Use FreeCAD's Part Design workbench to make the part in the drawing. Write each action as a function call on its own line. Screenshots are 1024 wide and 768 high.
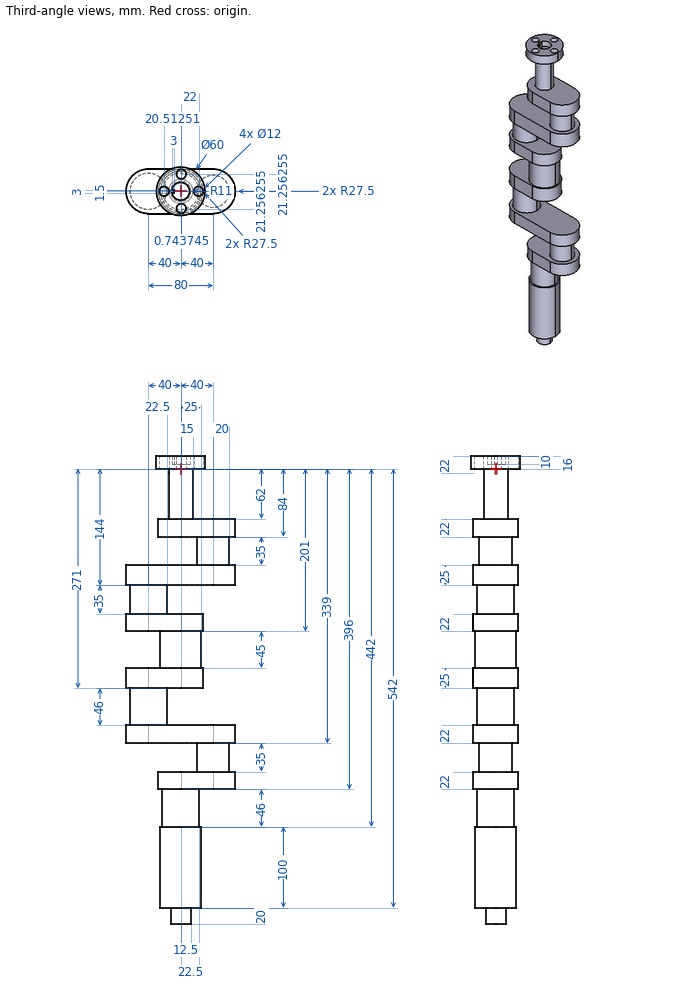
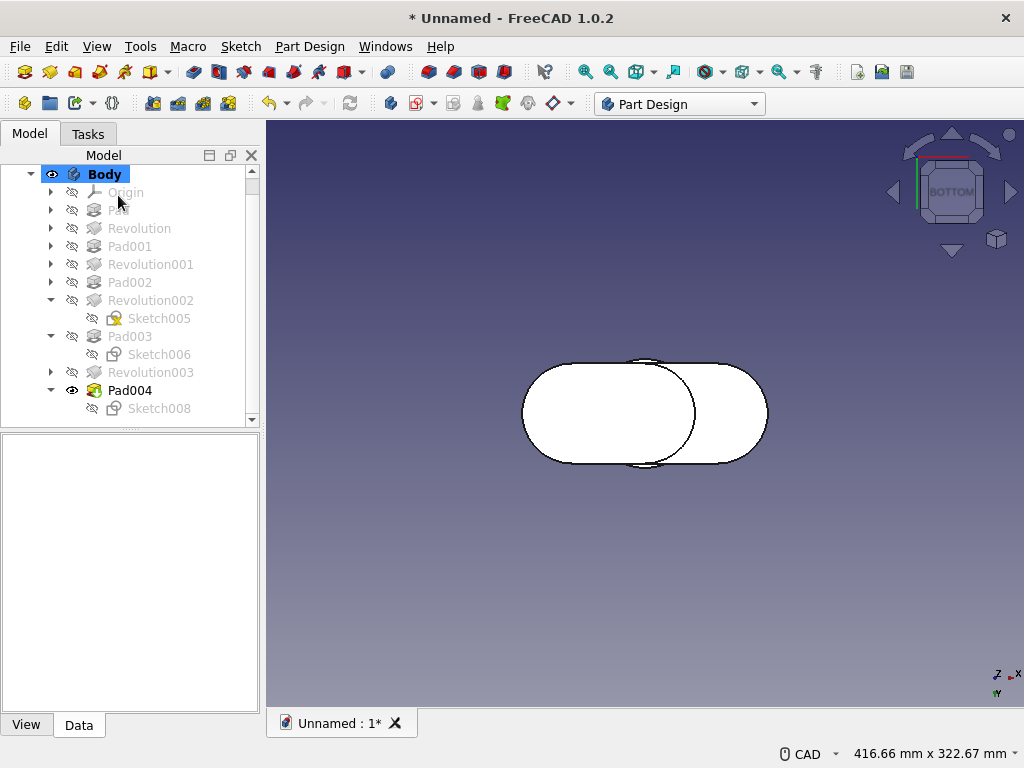
click(416, 104)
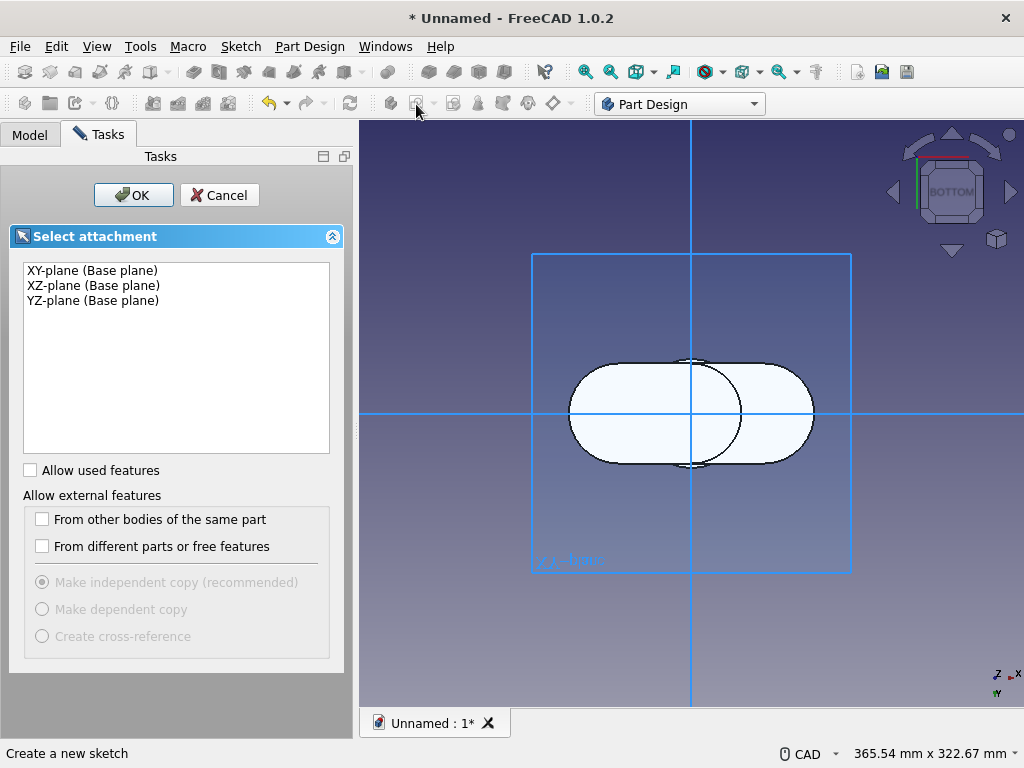
click(84, 286)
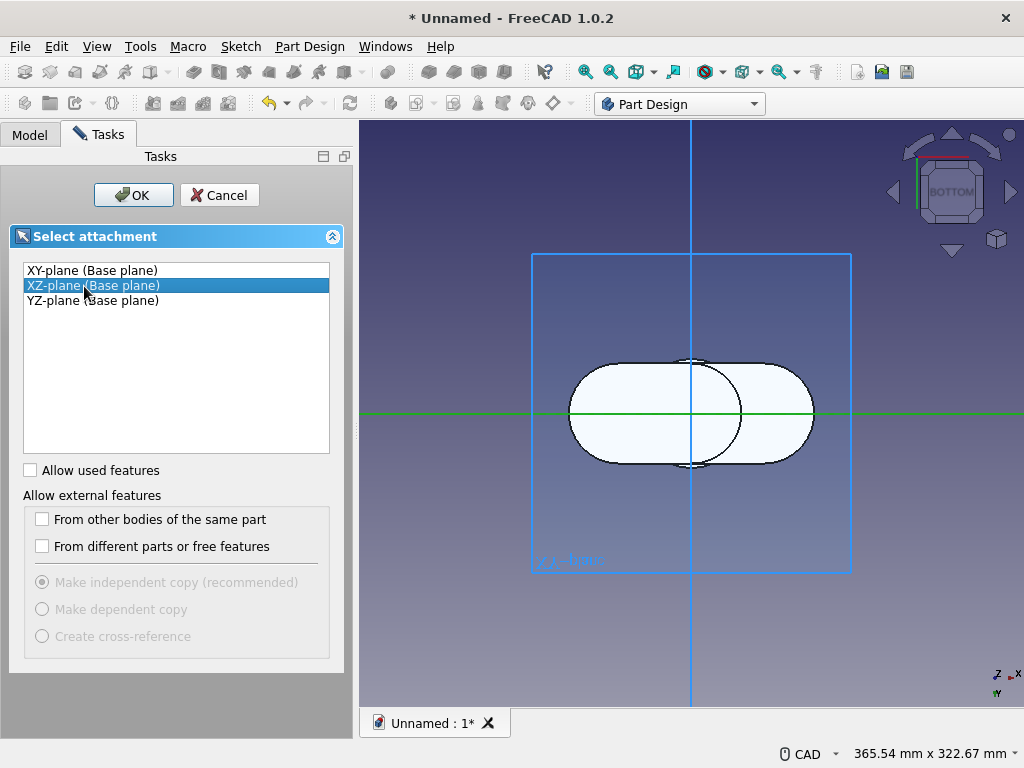
click(134, 195)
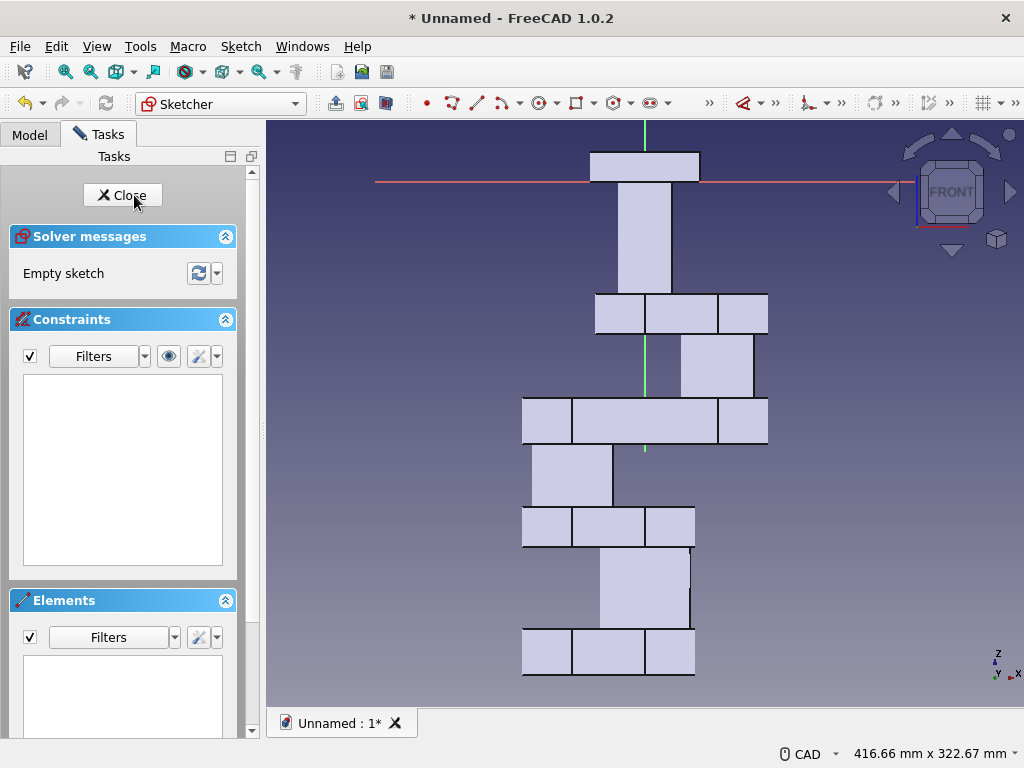
click(386, 104)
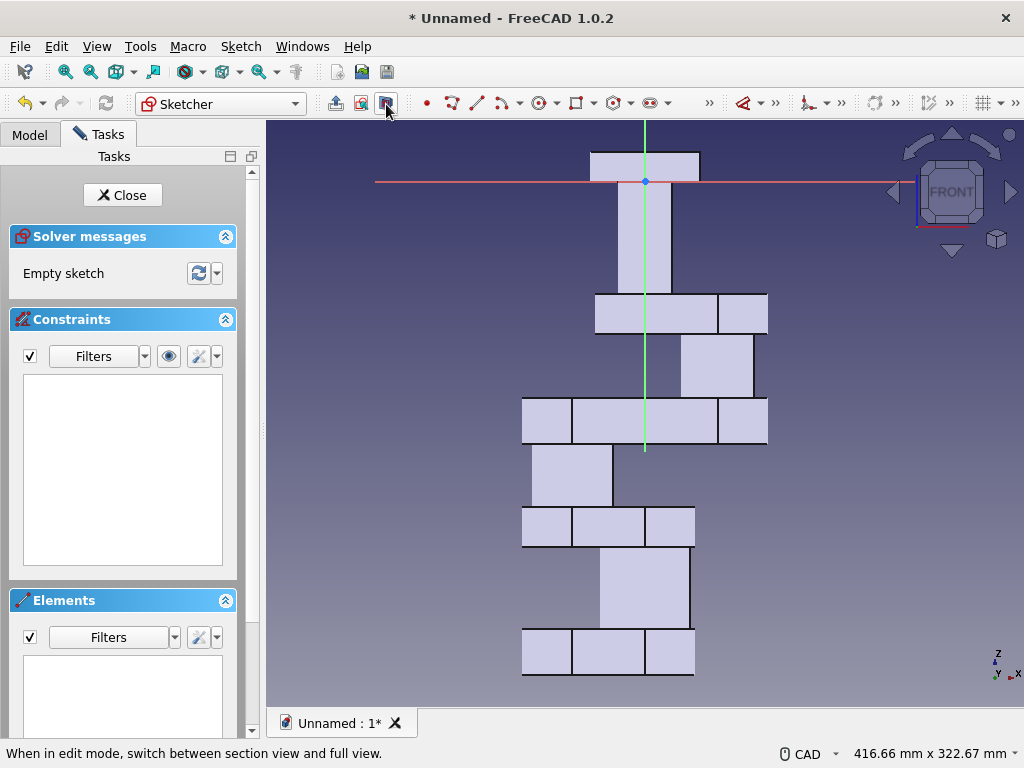
scroll(576, 414, down, 5)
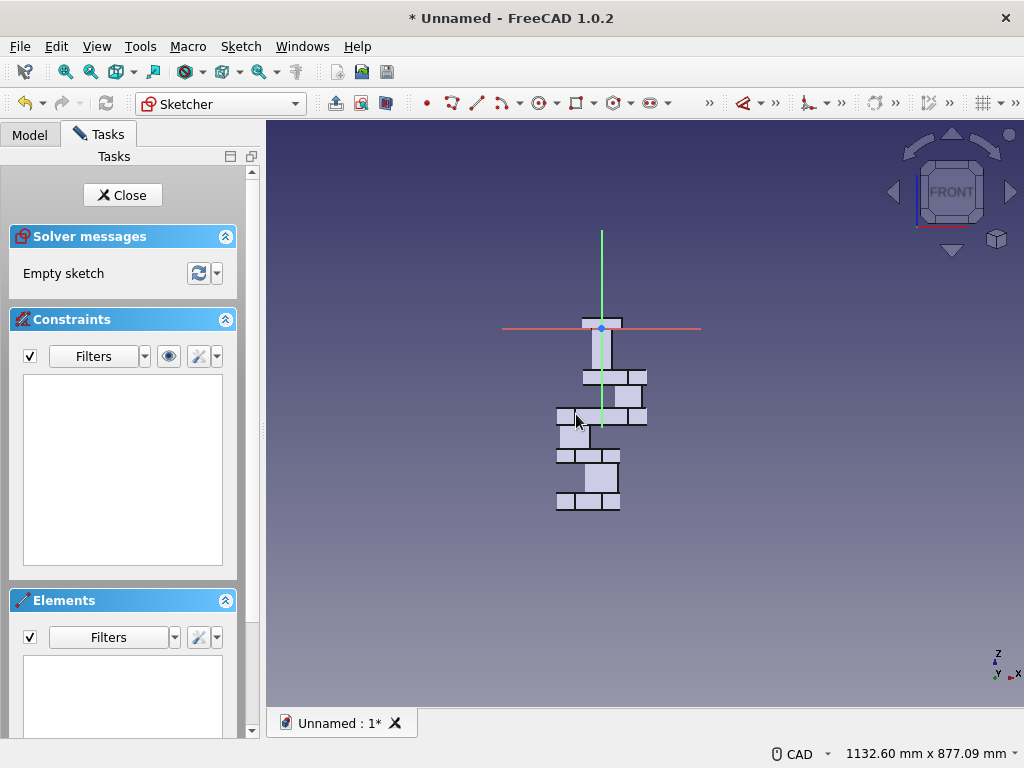
scroll(583, 546, up, 11)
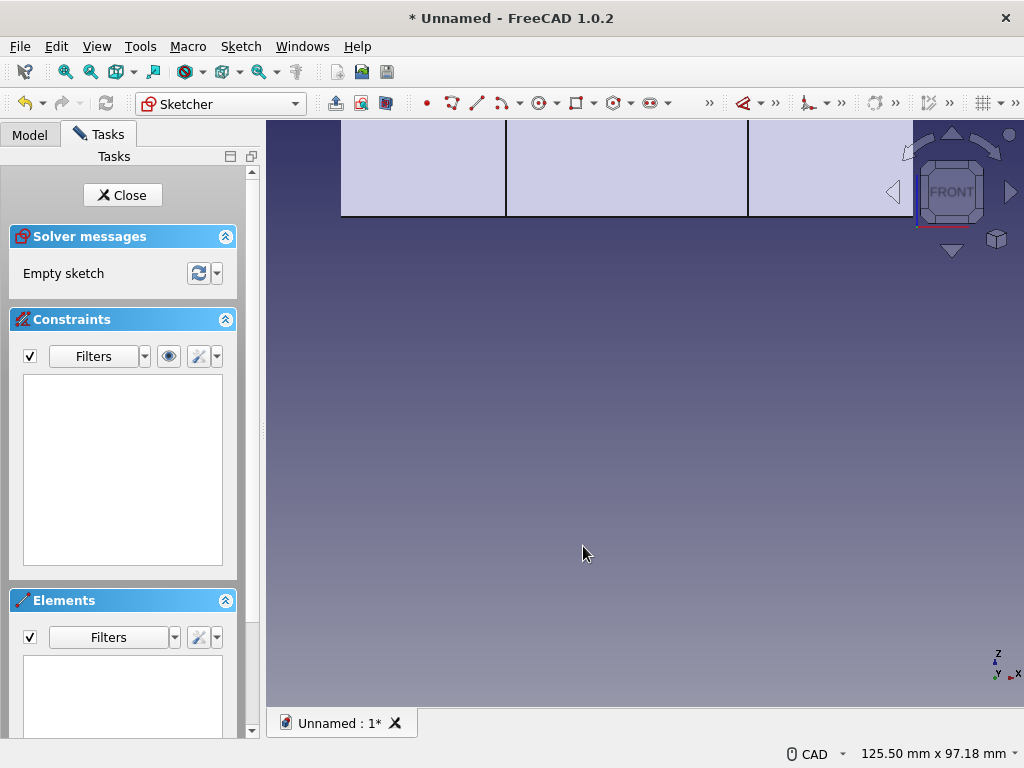
key(g)
key(r)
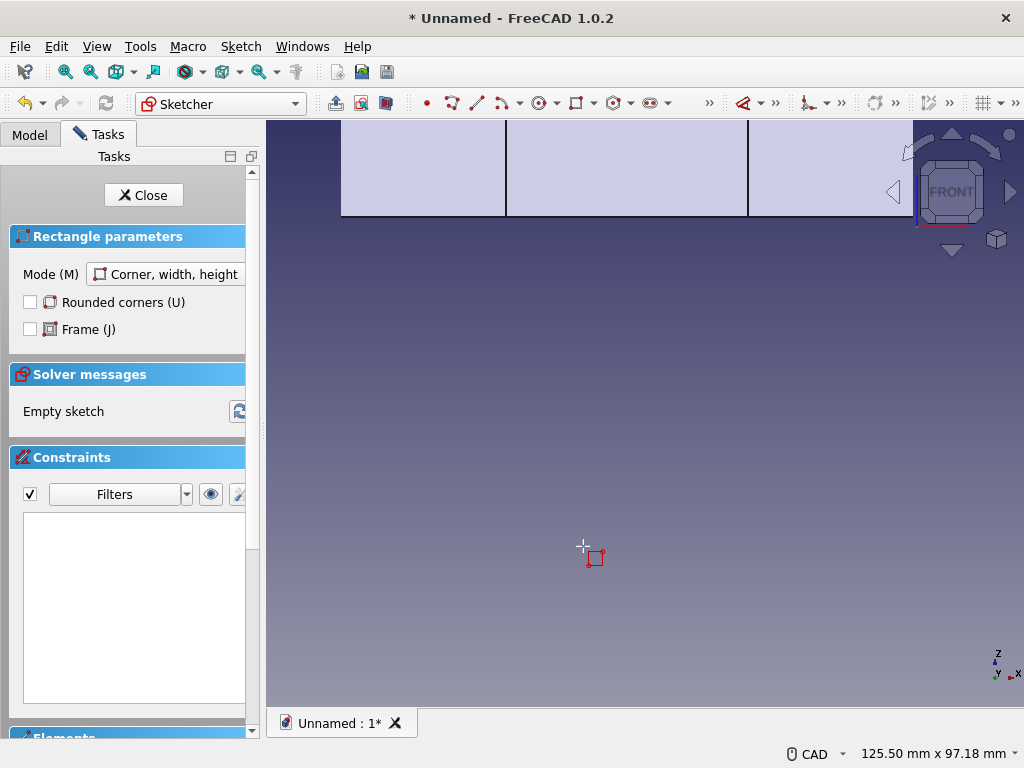
click(506, 217)
move(642, 495)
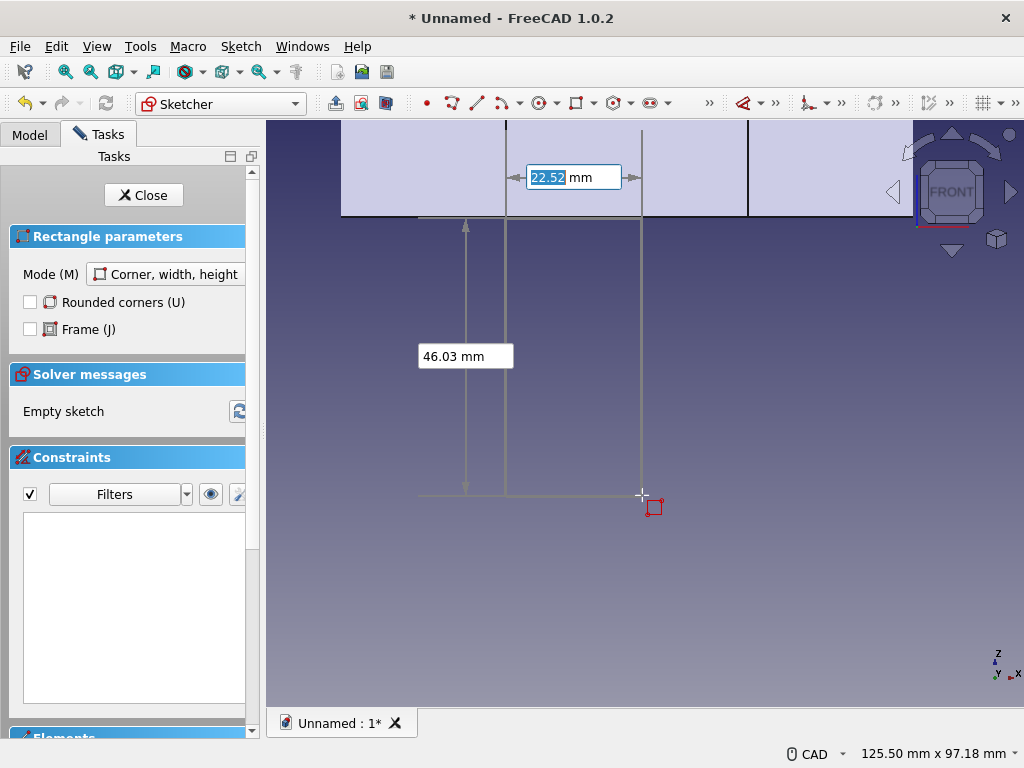
text(22.5)
key(Tab)
text(46)
key(Return)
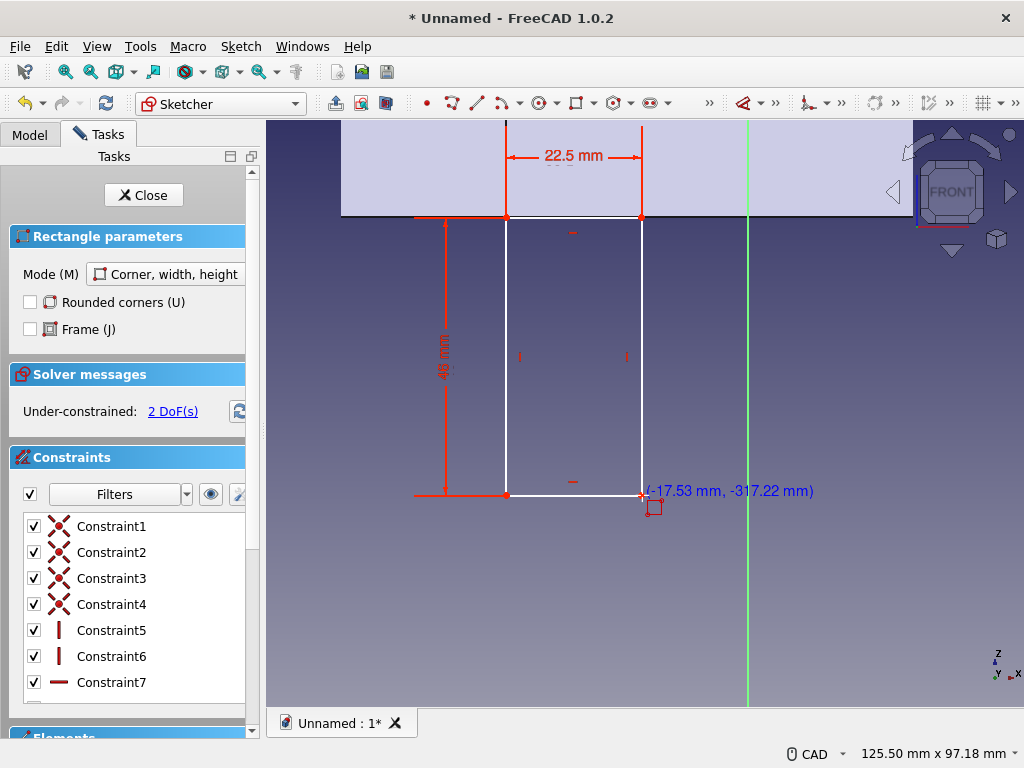
key(g)
key(l)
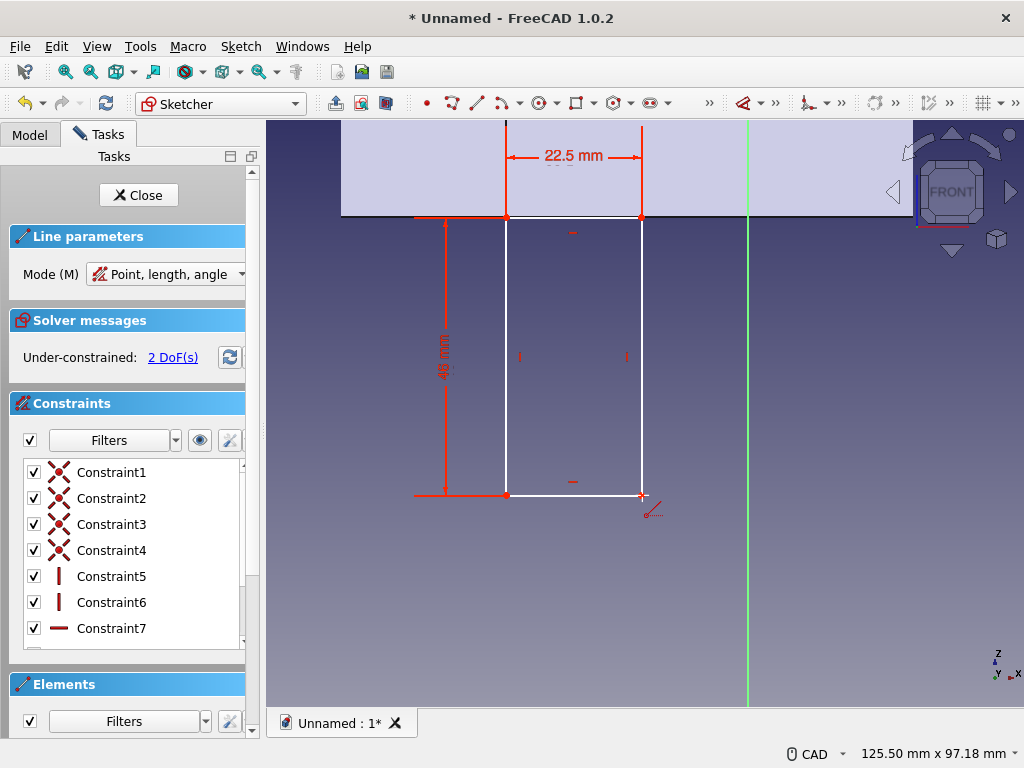
click(506, 522)
click(506, 606)
key(Escape)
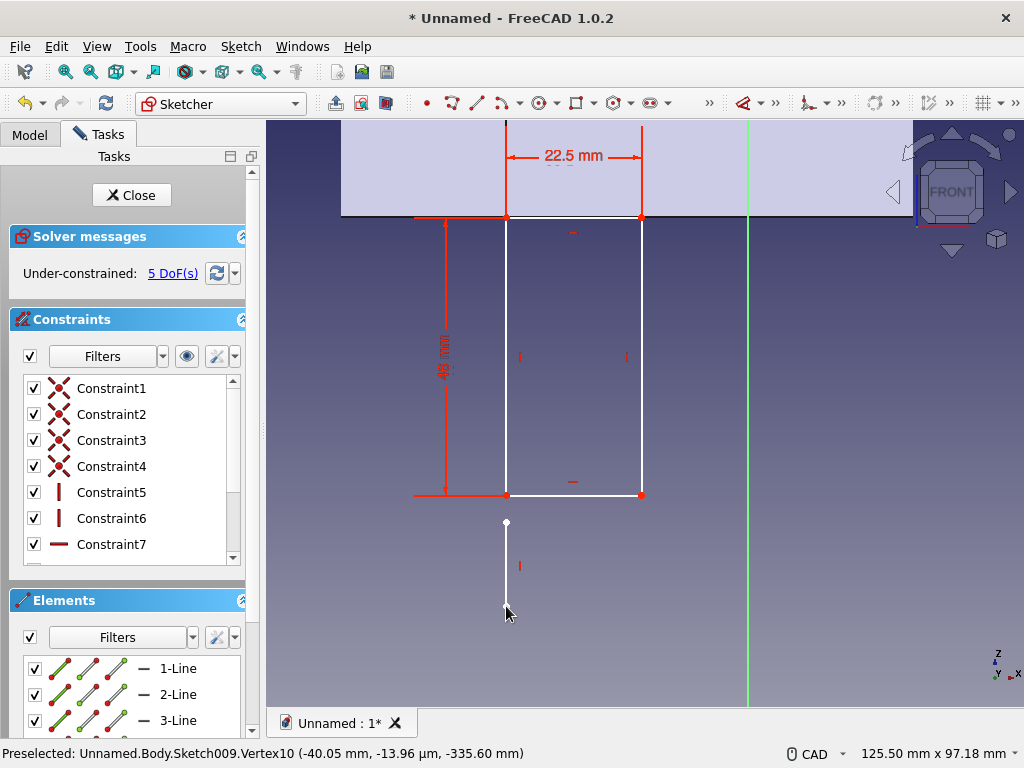
click(506, 548)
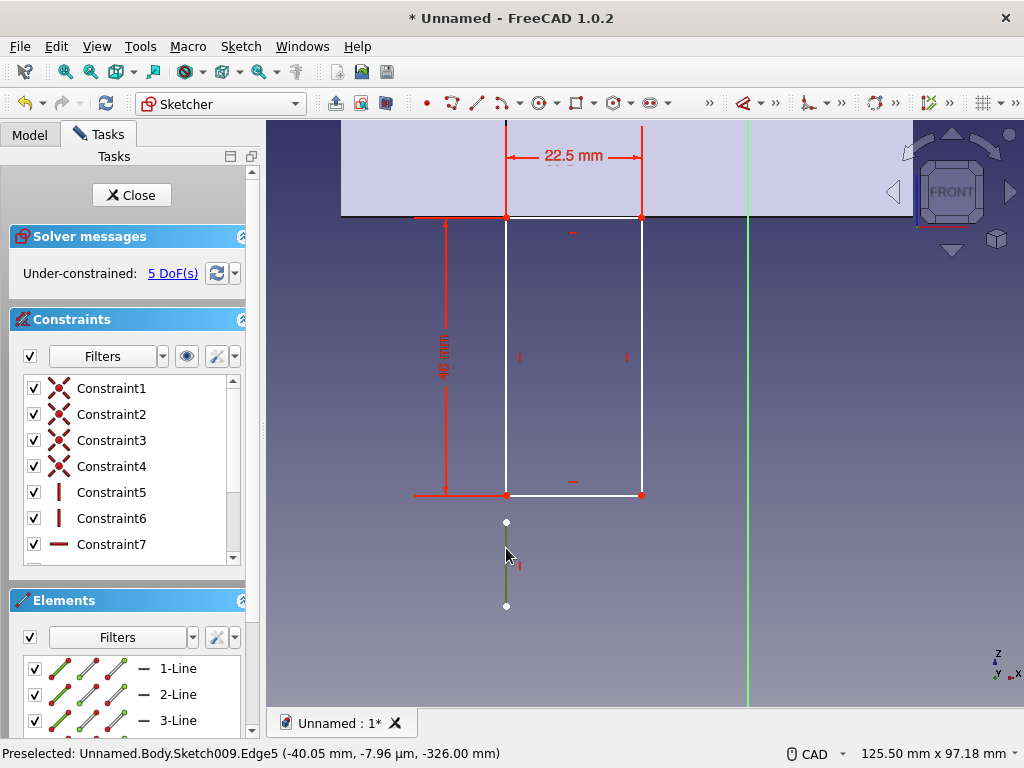
key(g)
key(n)